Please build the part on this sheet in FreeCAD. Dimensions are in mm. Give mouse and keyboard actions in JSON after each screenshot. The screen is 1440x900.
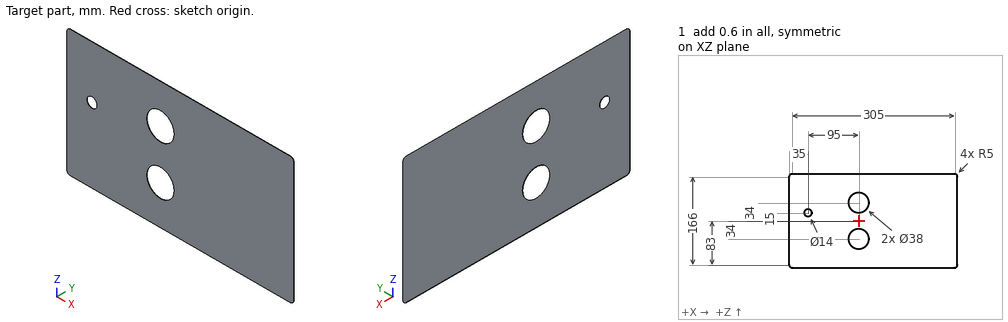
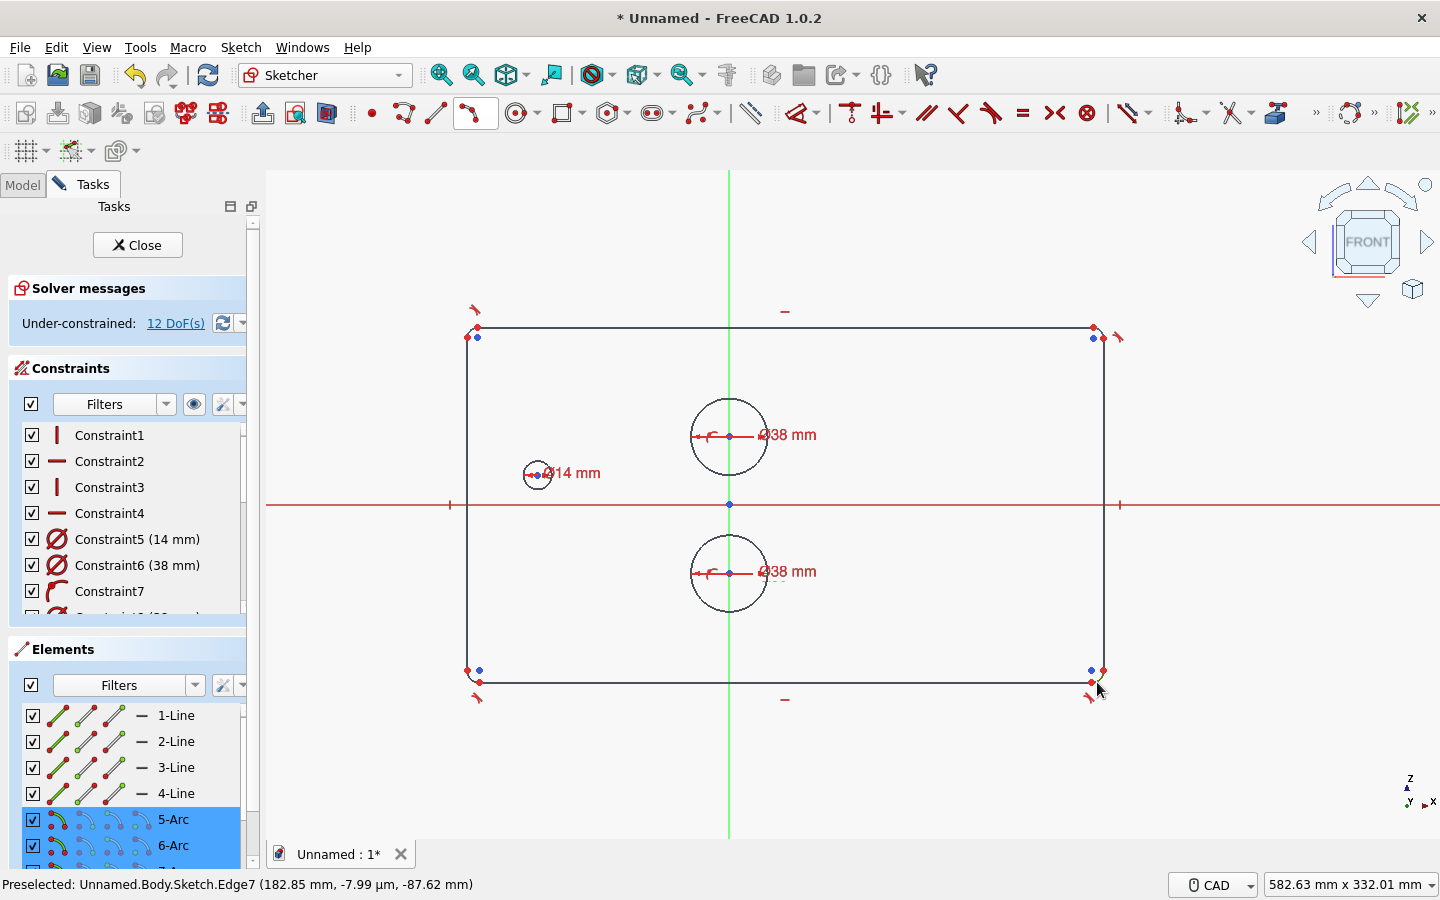
{"action": "scroll", "coordinate": [469, 676], "scroll_direction": "up", "scroll_amount": 5}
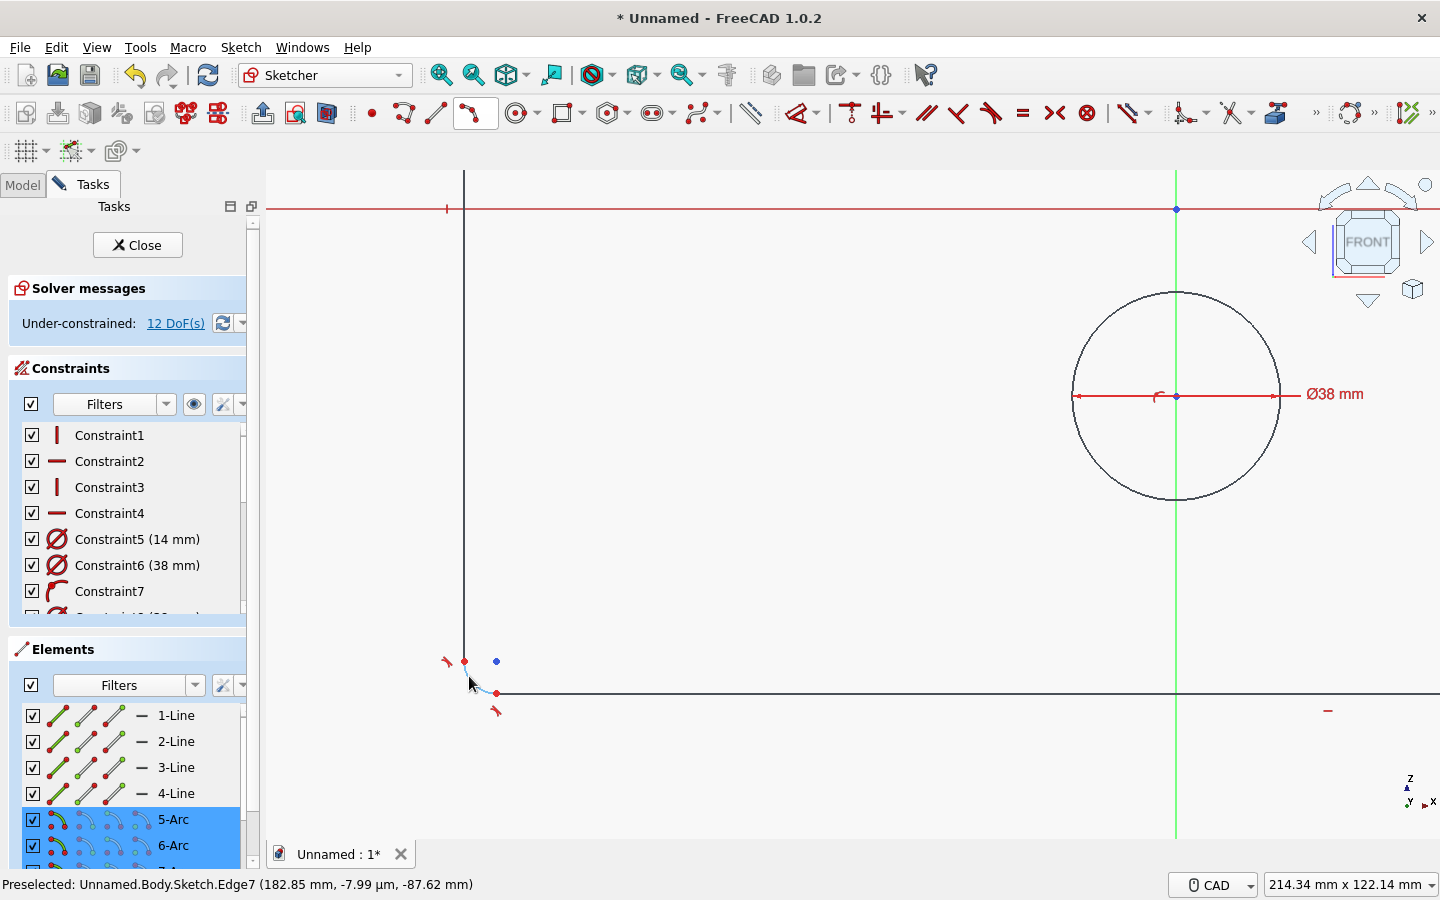
{"action": "left_click", "coordinate": [468, 676]}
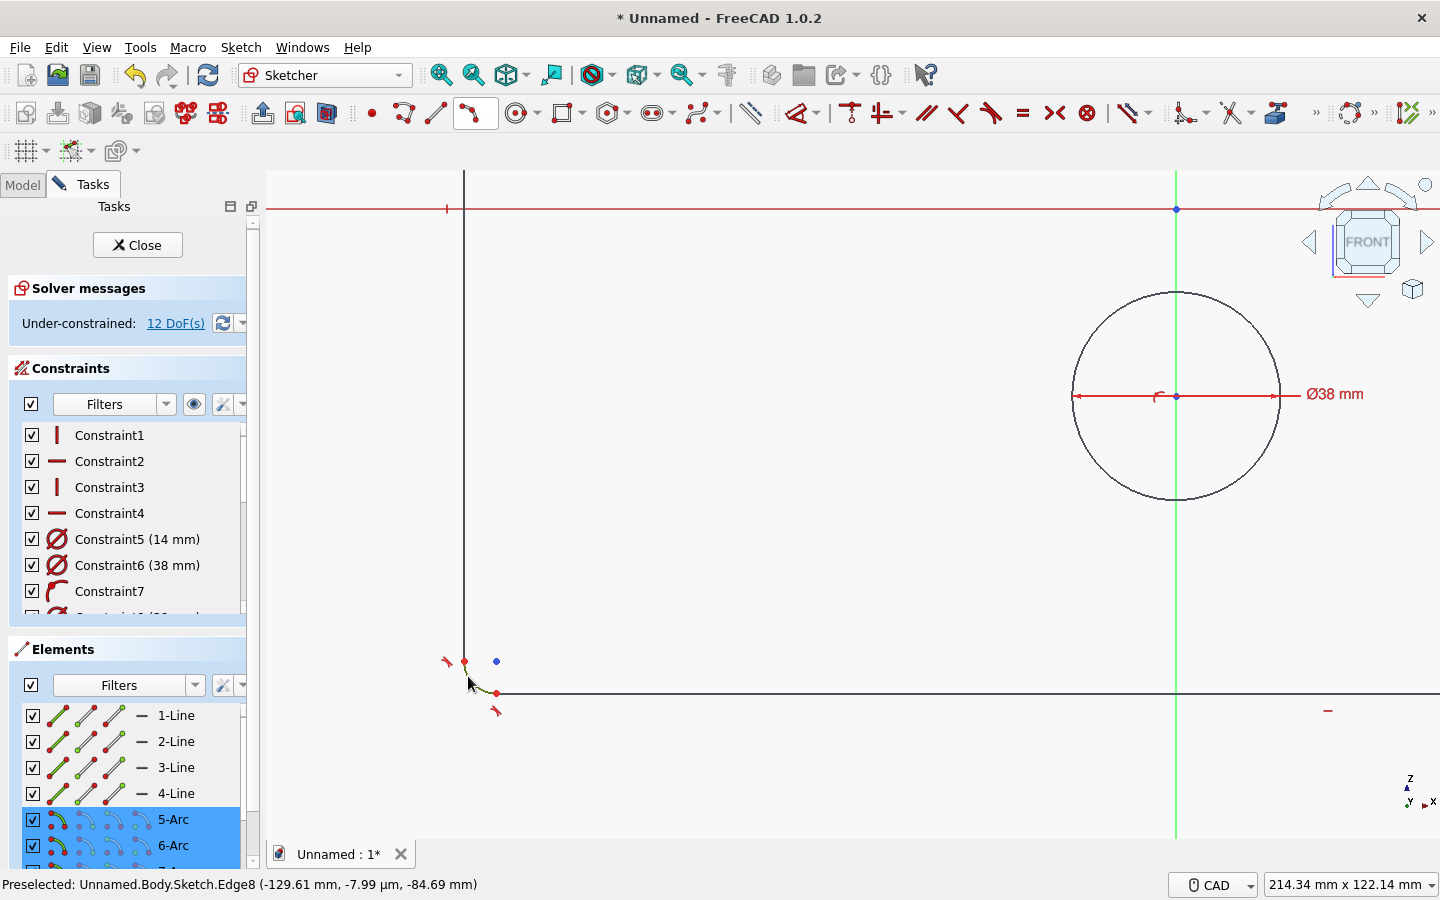
{"action": "left_click", "coordinate": [1024, 114]}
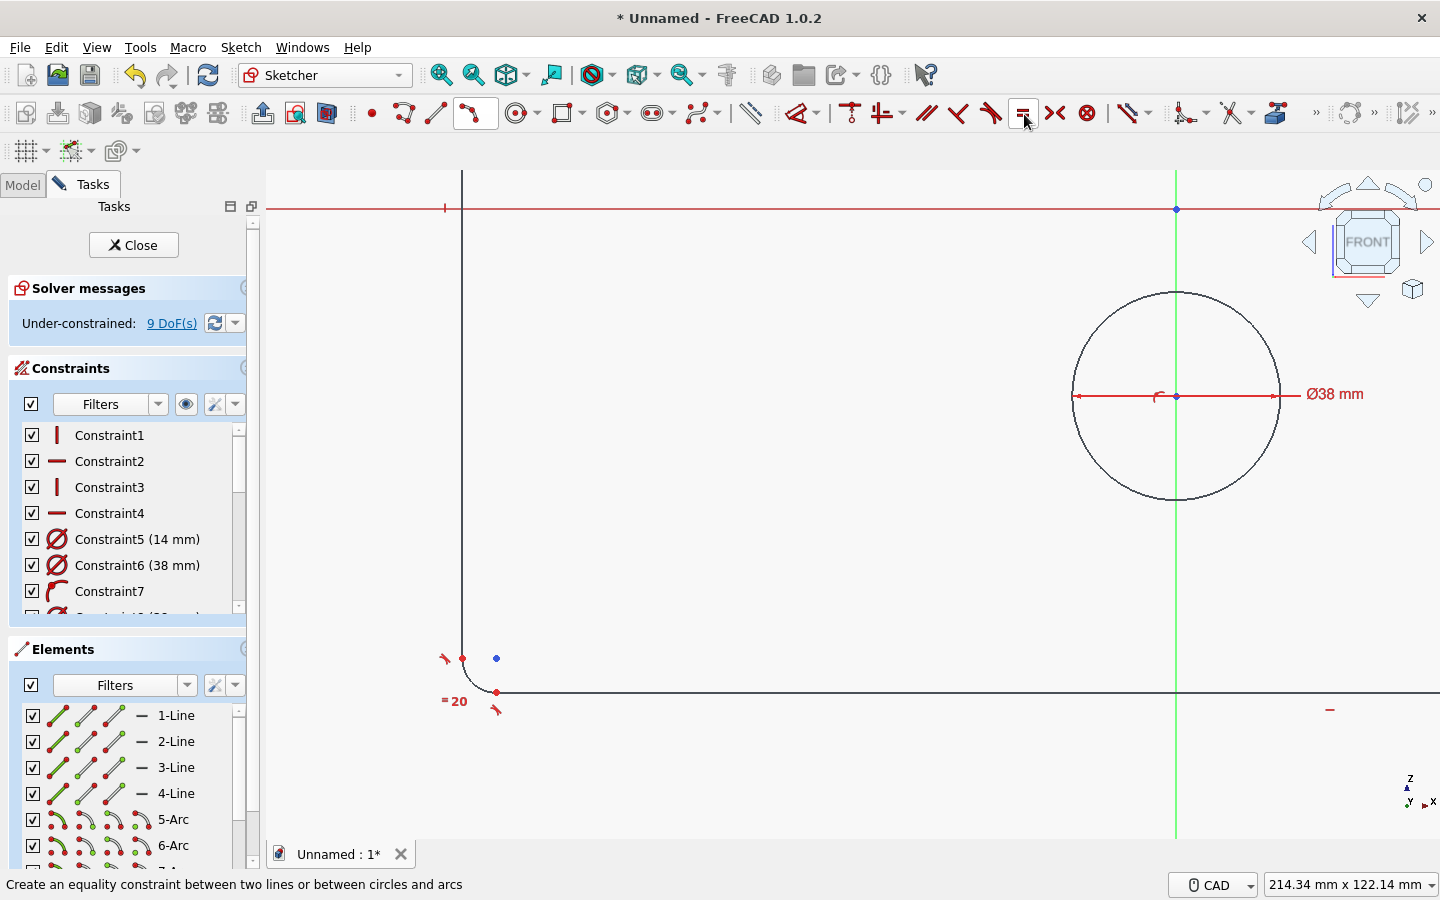
{"action": "scroll", "coordinate": [469, 676], "scroll_direction": "down", "scroll_amount": 5}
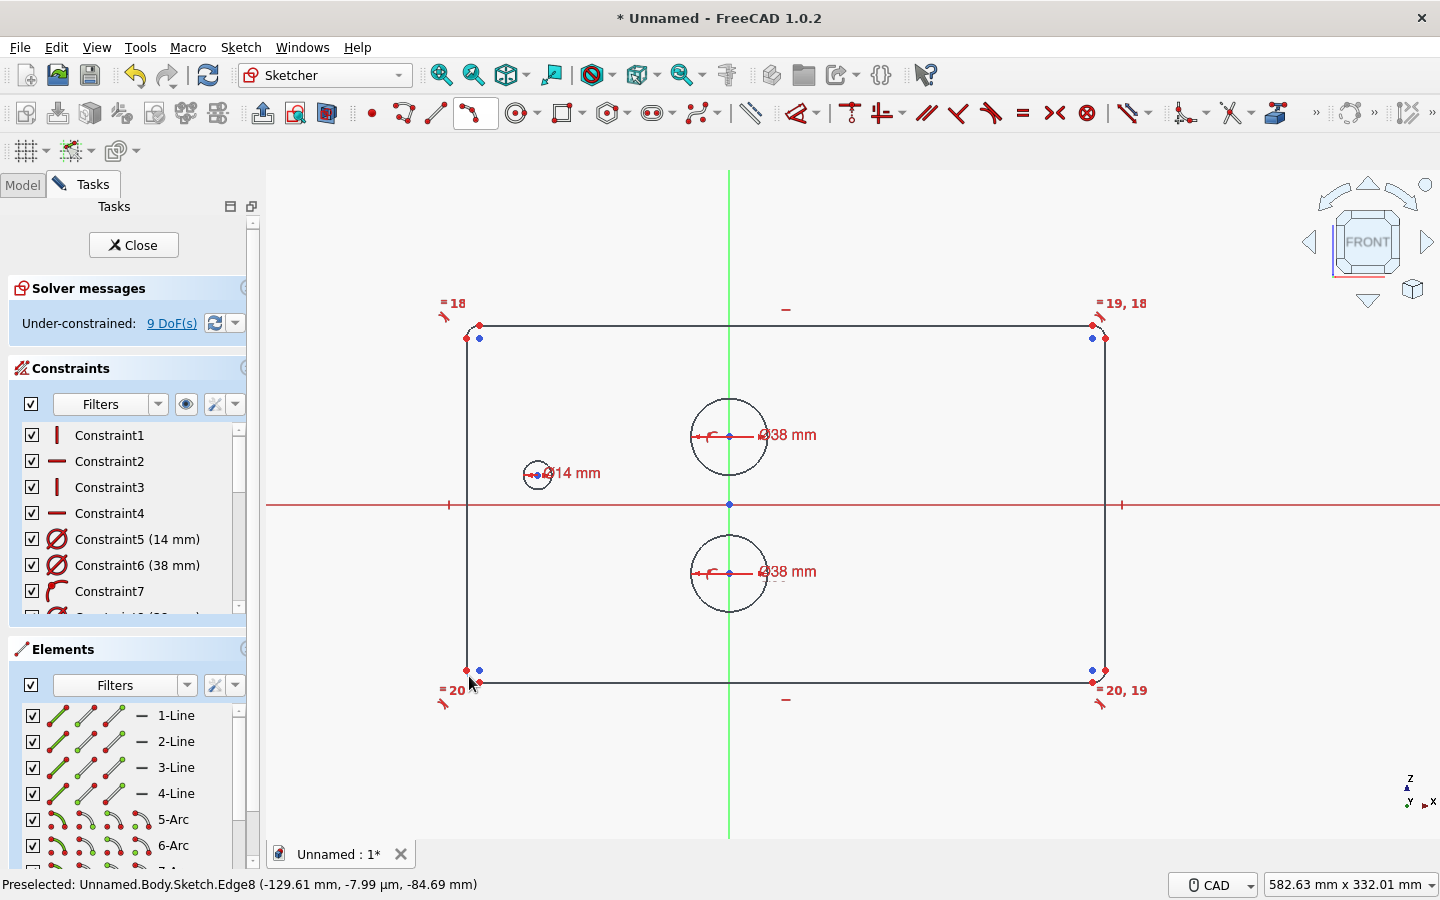
{"action": "scroll", "coordinate": [474, 327], "scroll_direction": "up", "scroll_amount": 7}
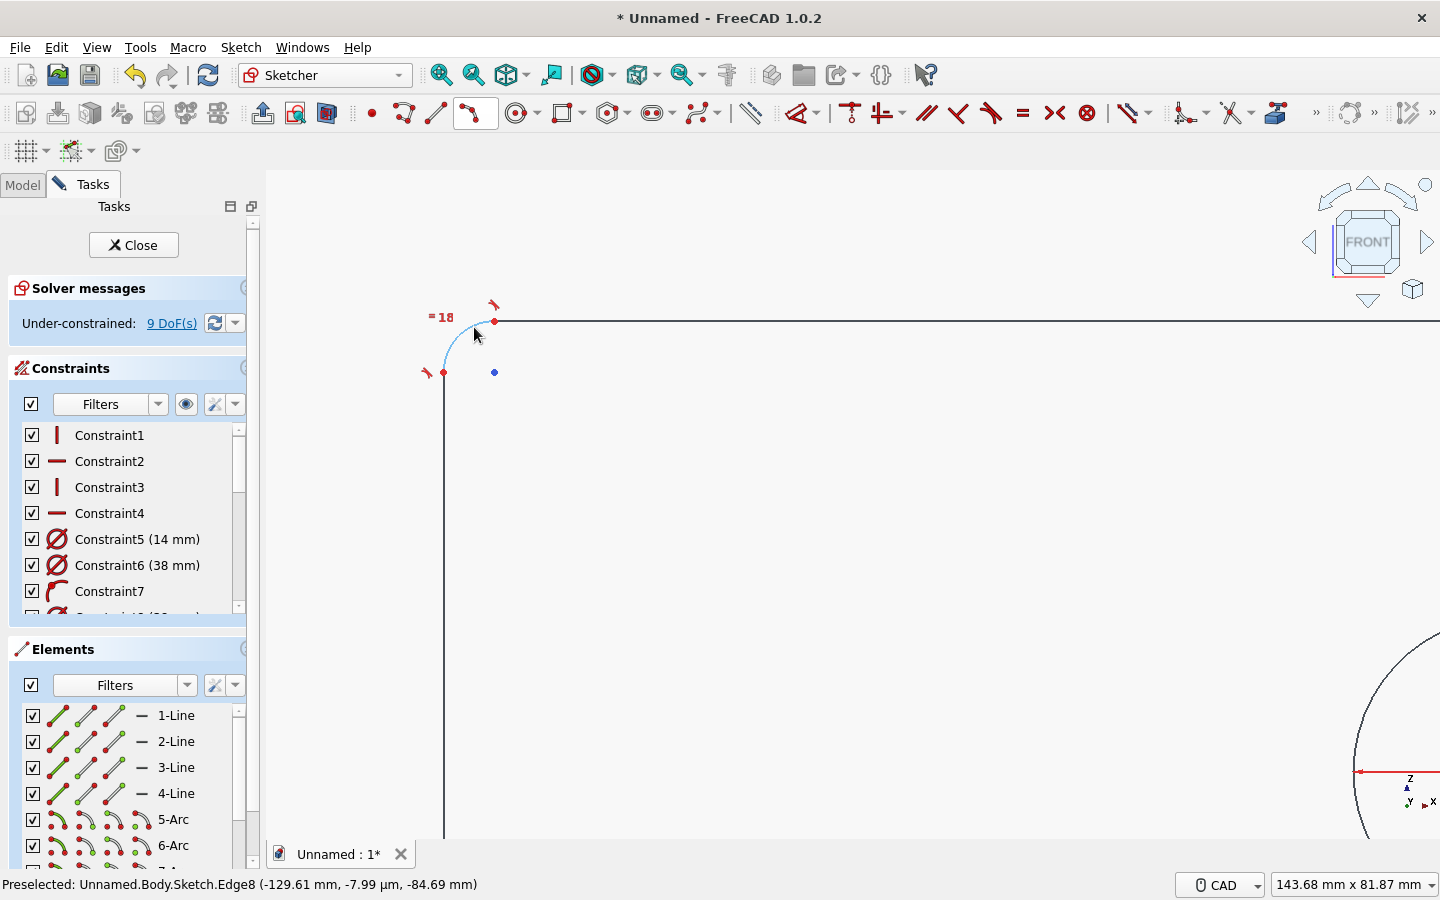
{"action": "left_click", "coordinate": [472, 327]}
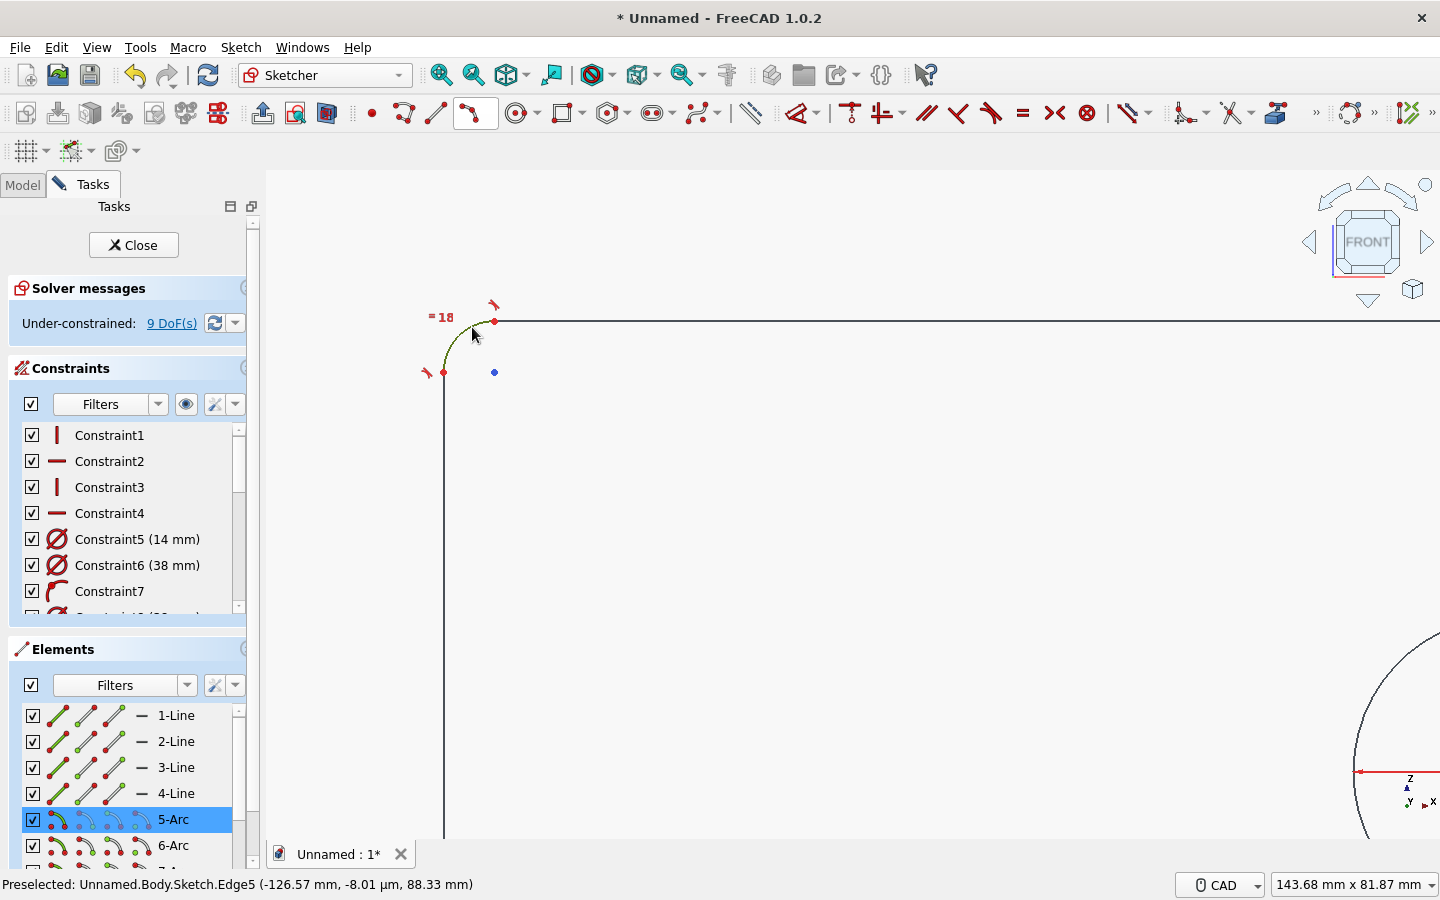
{"action": "left_click", "coordinate": [818, 114]}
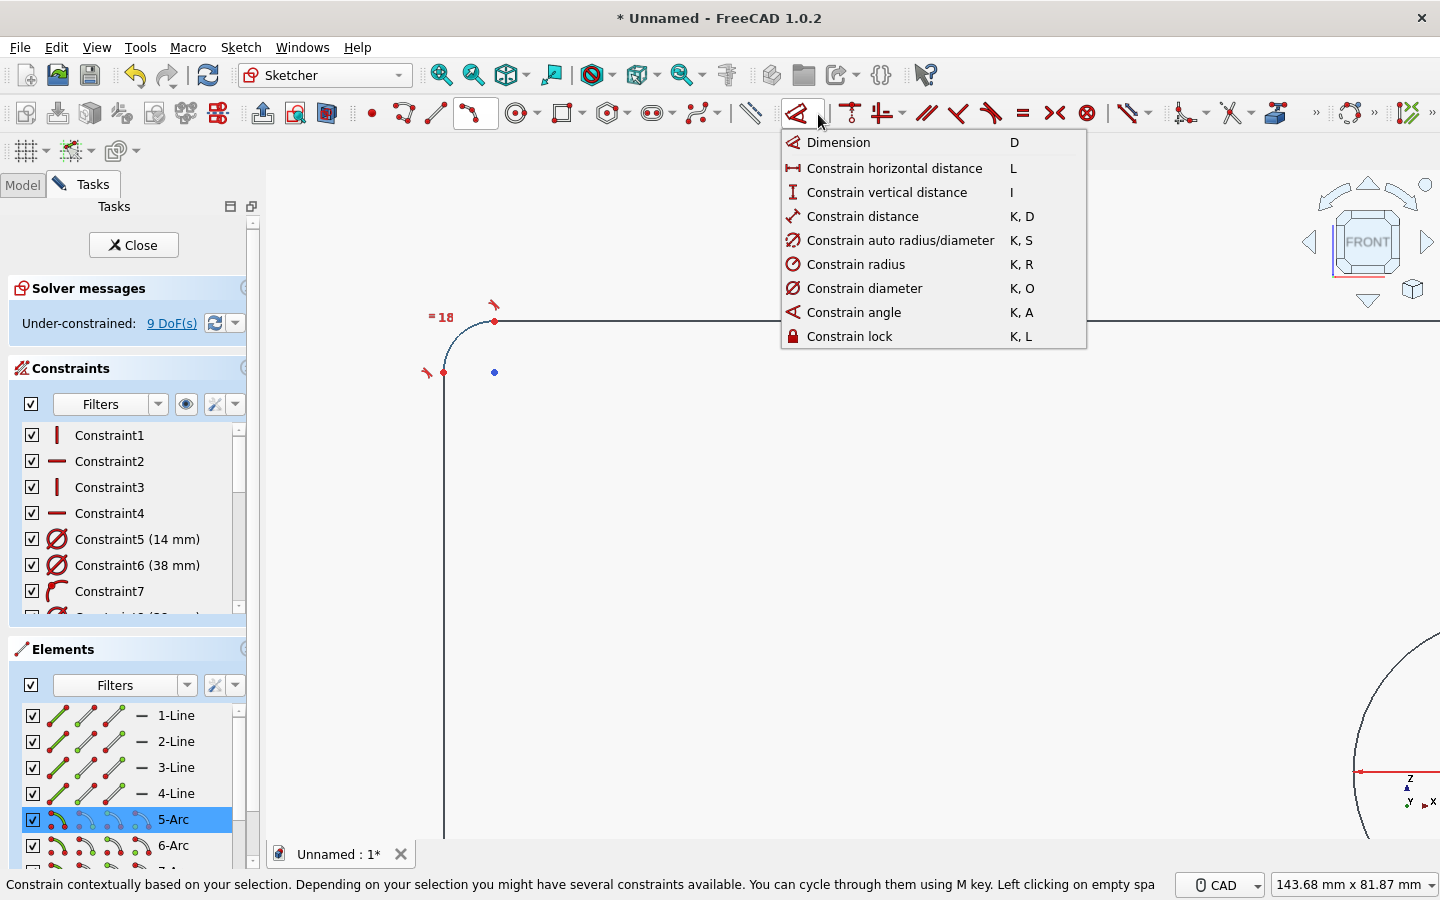
{"action": "left_click", "coordinate": [934, 264]}